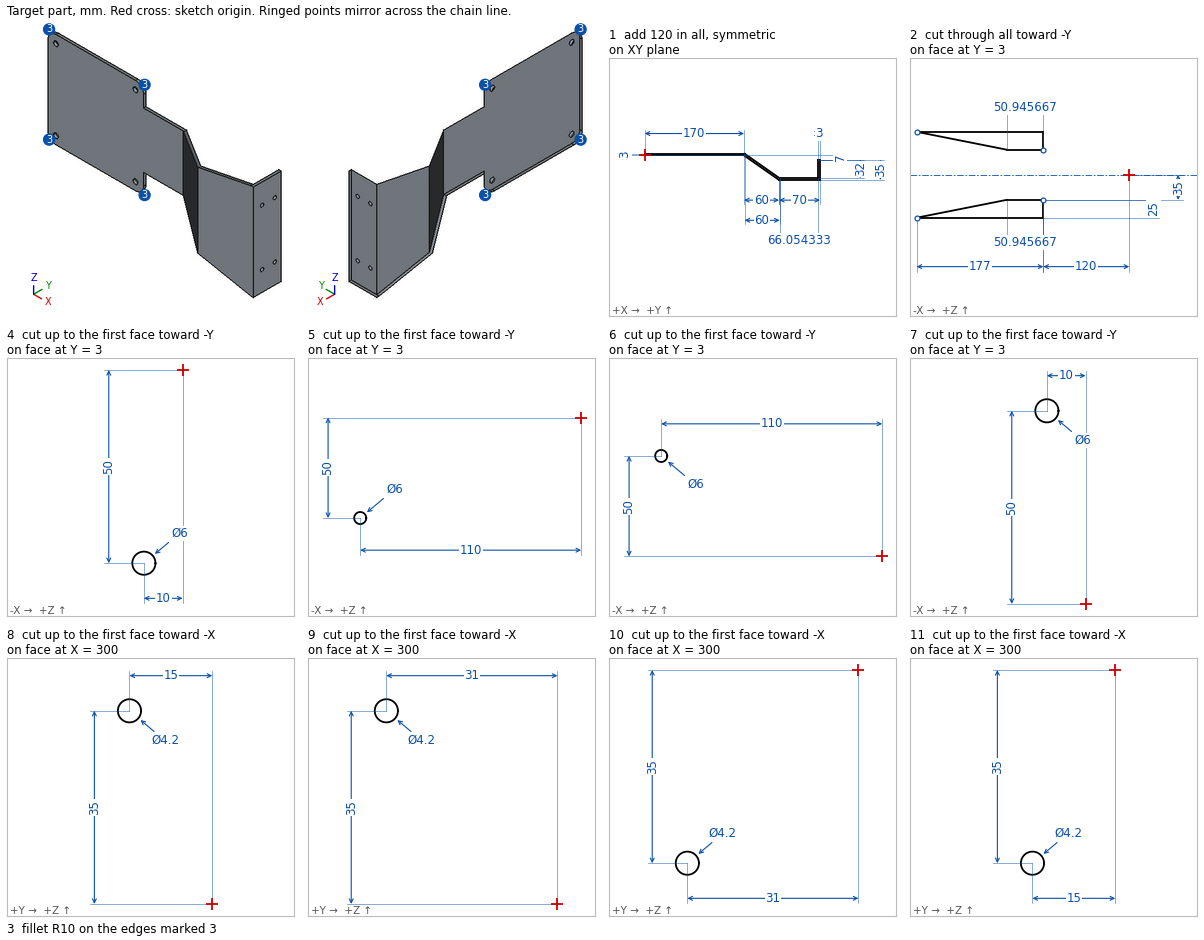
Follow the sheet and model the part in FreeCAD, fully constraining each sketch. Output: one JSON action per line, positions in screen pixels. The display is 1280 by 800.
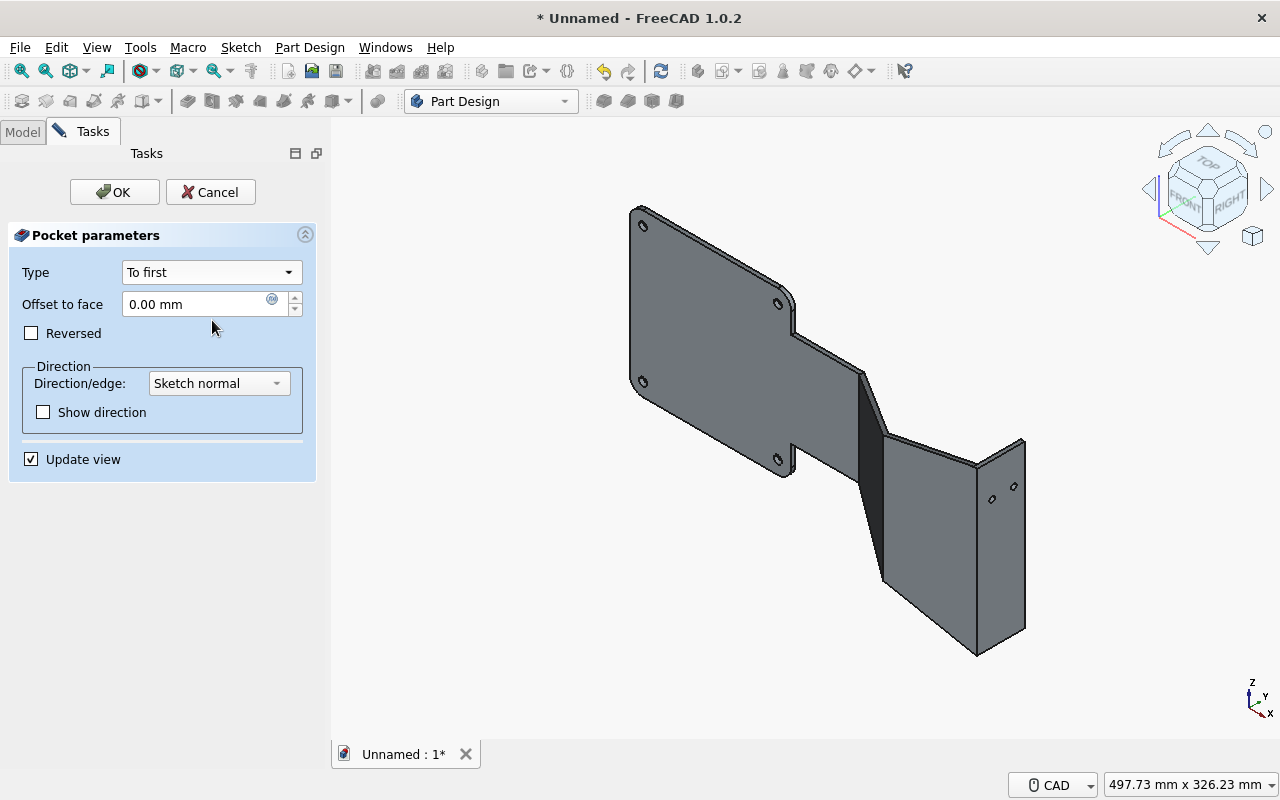
{"action": "left_click", "coordinate": [115, 192]}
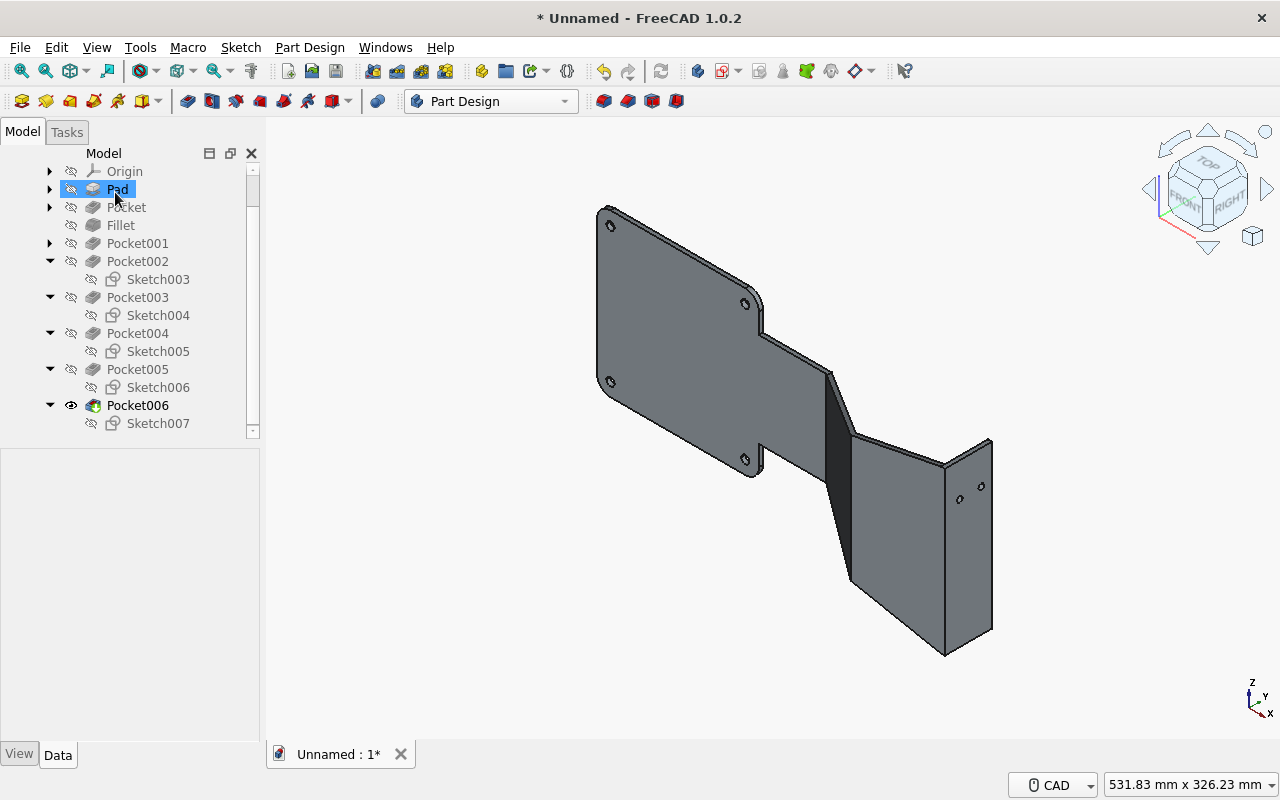
{"action": "left_click", "coordinate": [968, 548]}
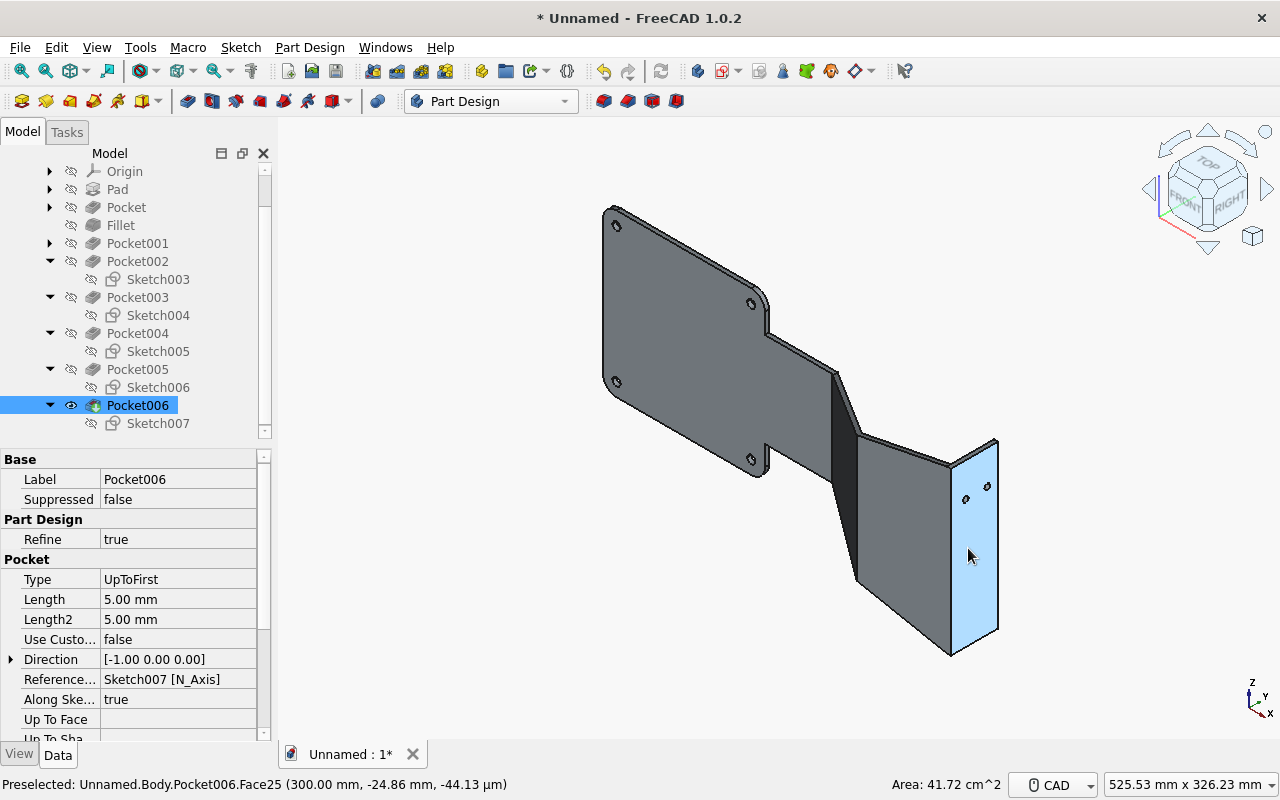
{"action": "left_click", "coordinate": [722, 72]}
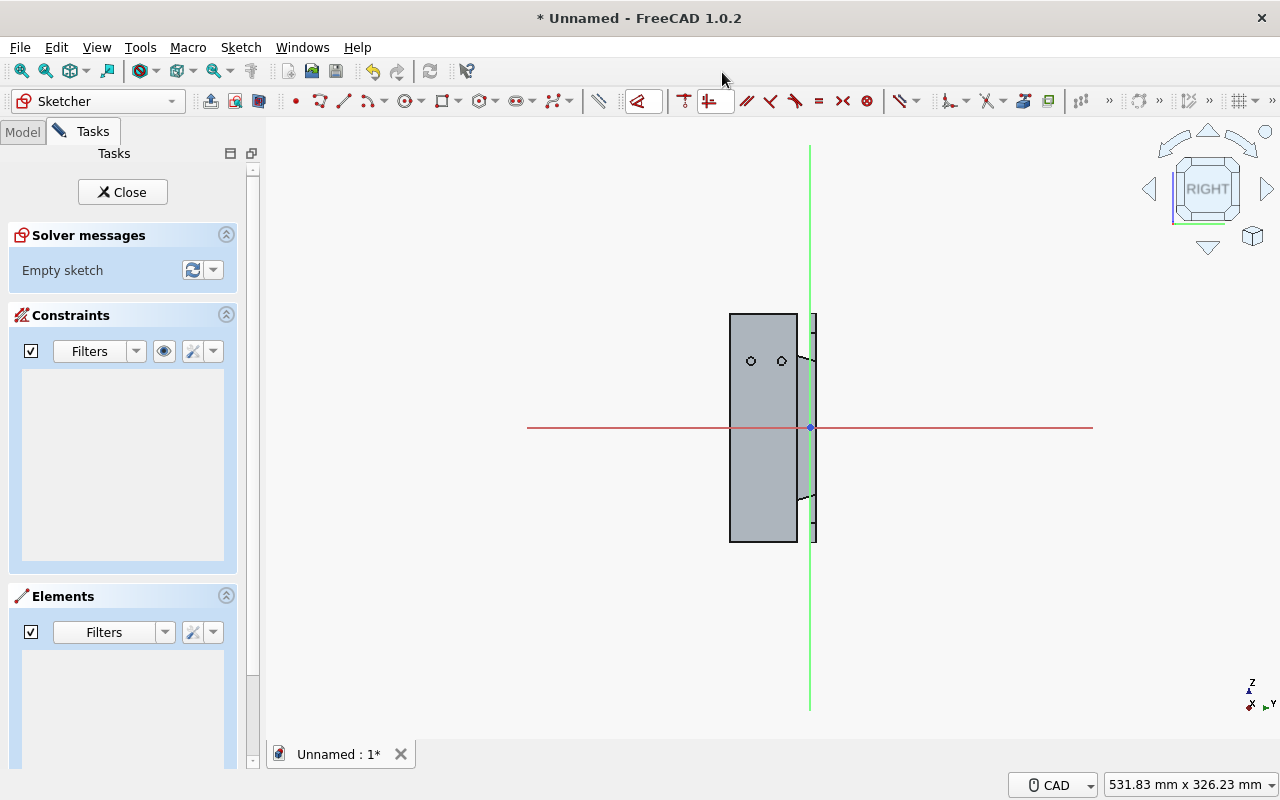
{"action": "scroll", "coordinate": [754, 498], "scroll_direction": "up", "scroll_amount": 15}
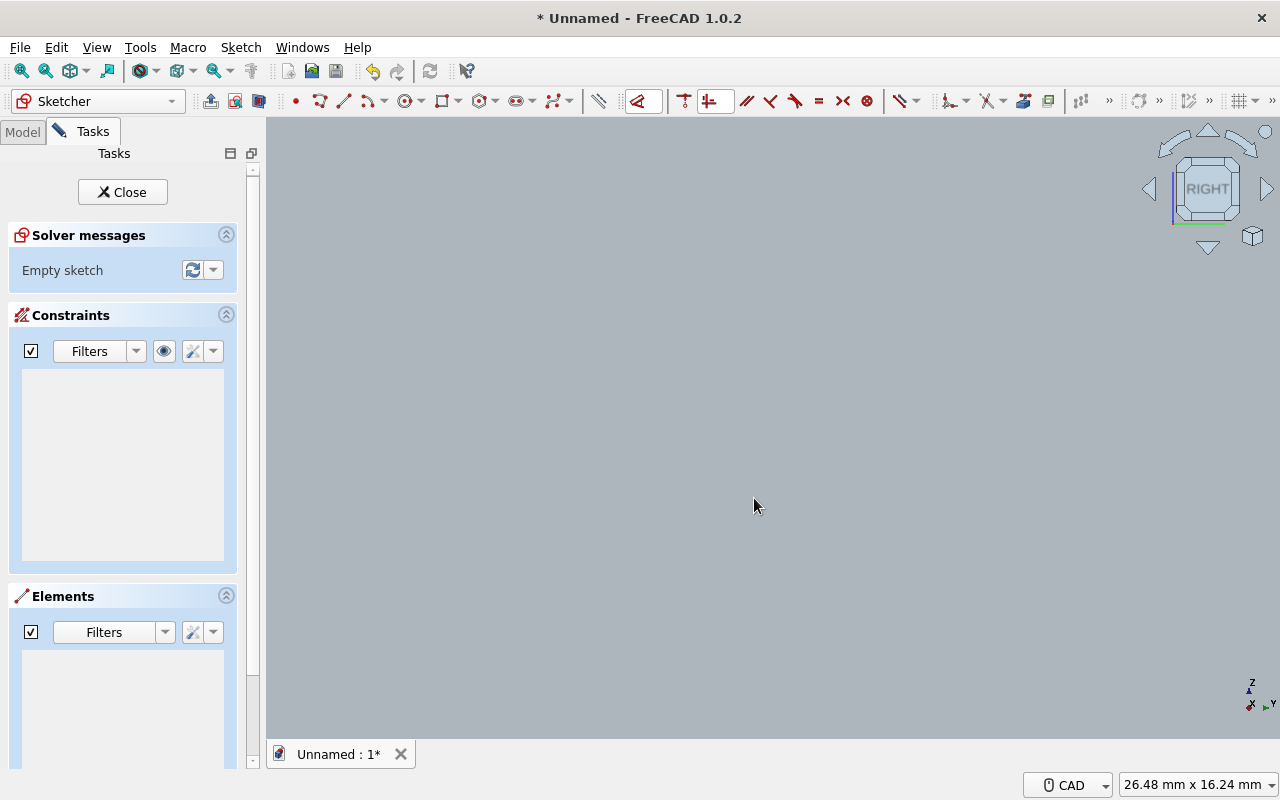
{"action": "scroll", "coordinate": [675, 416], "scroll_direction": "up", "scroll_amount": 5}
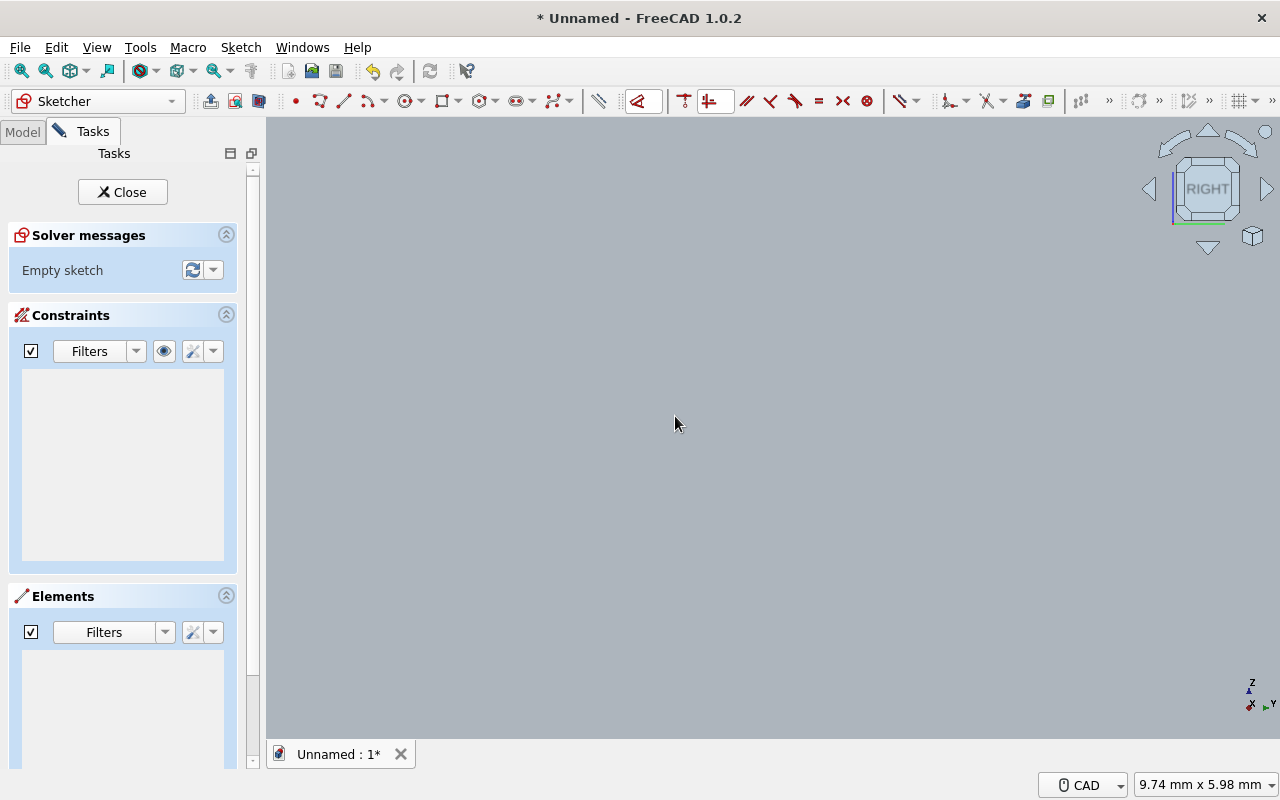
{"action": "left_click", "coordinate": [406, 102]}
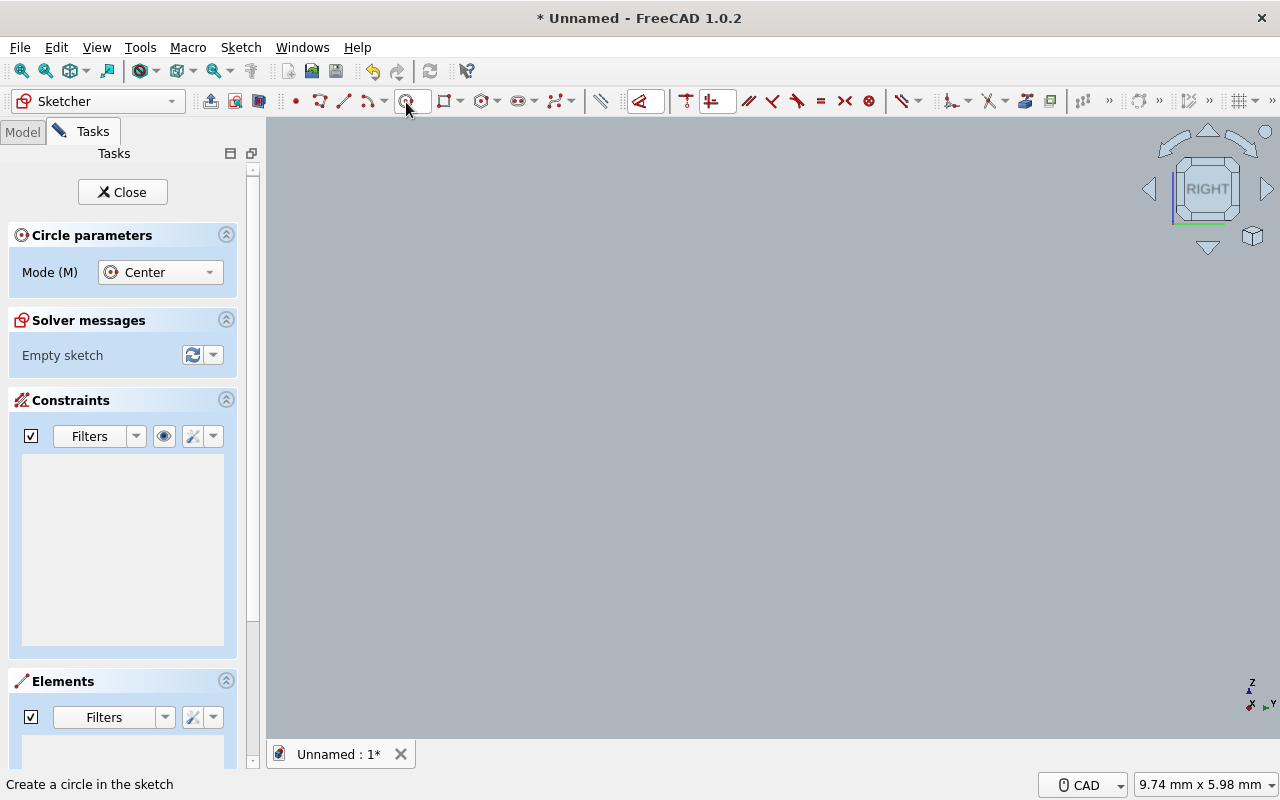
{"action": "left_click", "coordinate": [704, 428]}
{"action": "left_click", "coordinate": [859, 273]}
{"action": "key", "text": "Escape"}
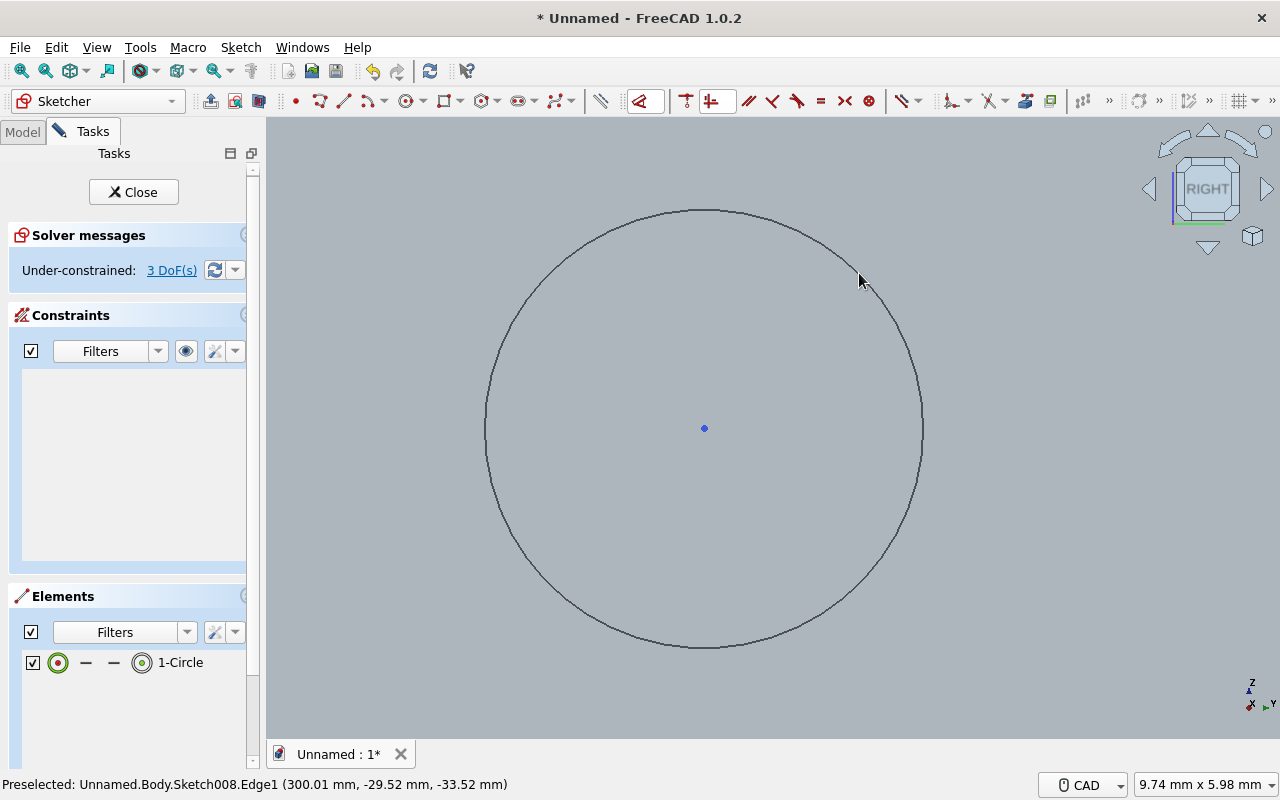
{"action": "left_click", "coordinate": [859, 274]}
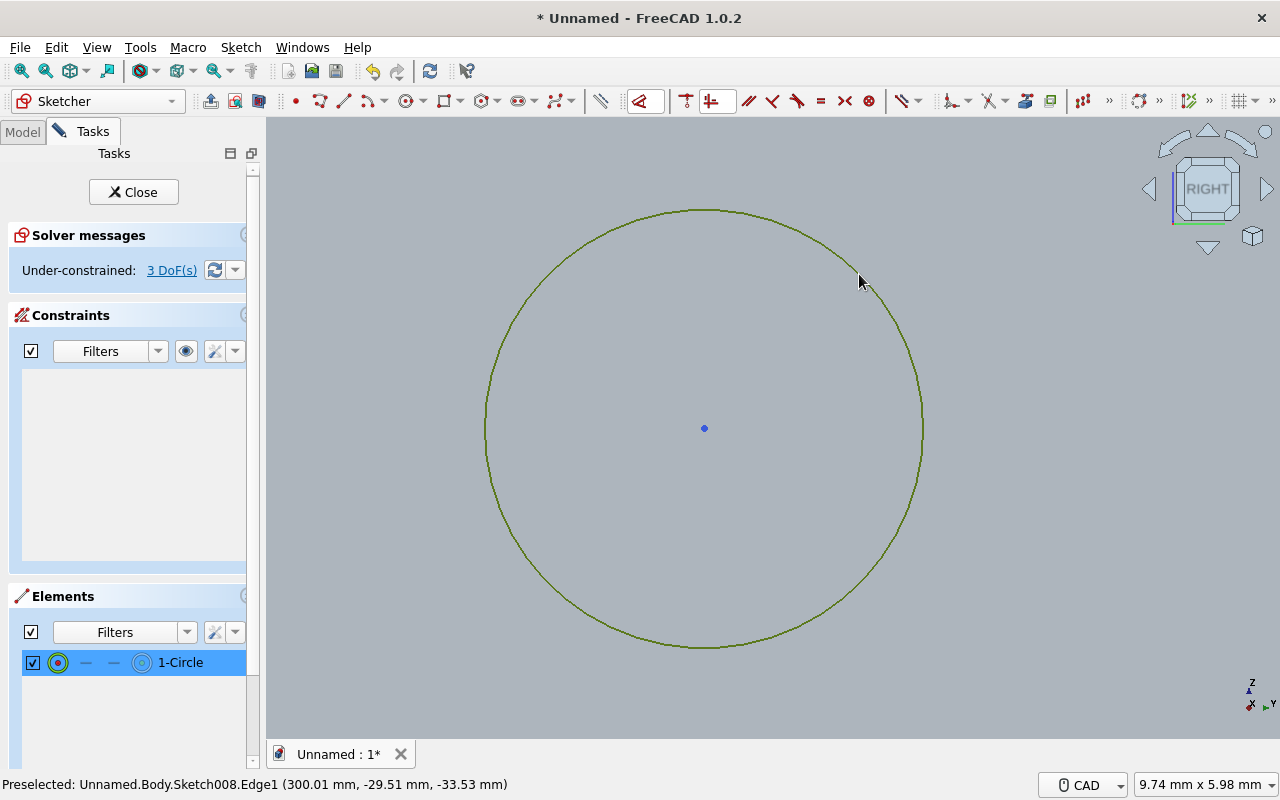
{"action": "key", "text": "k o"}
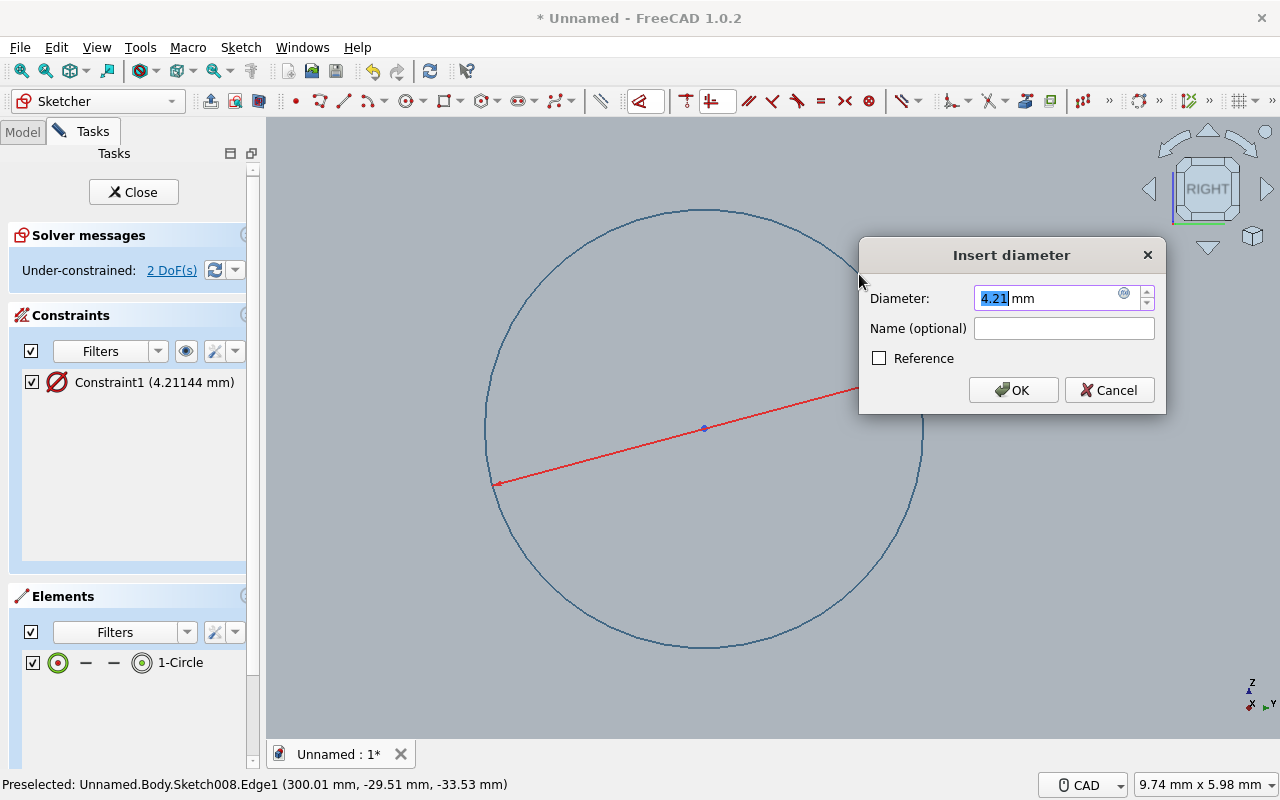
{"action": "type", "text": "4.2"}
{"action": "key", "text": "Return"}